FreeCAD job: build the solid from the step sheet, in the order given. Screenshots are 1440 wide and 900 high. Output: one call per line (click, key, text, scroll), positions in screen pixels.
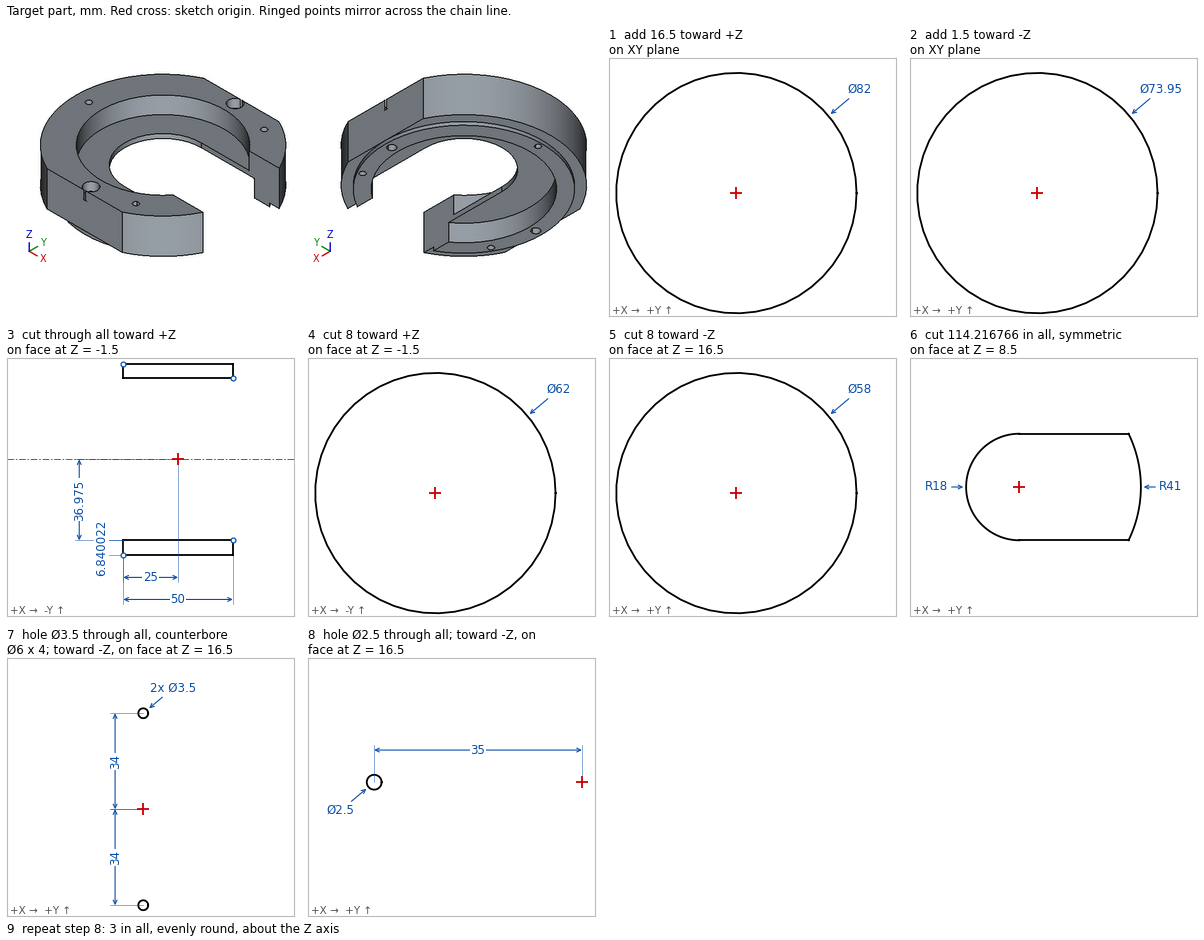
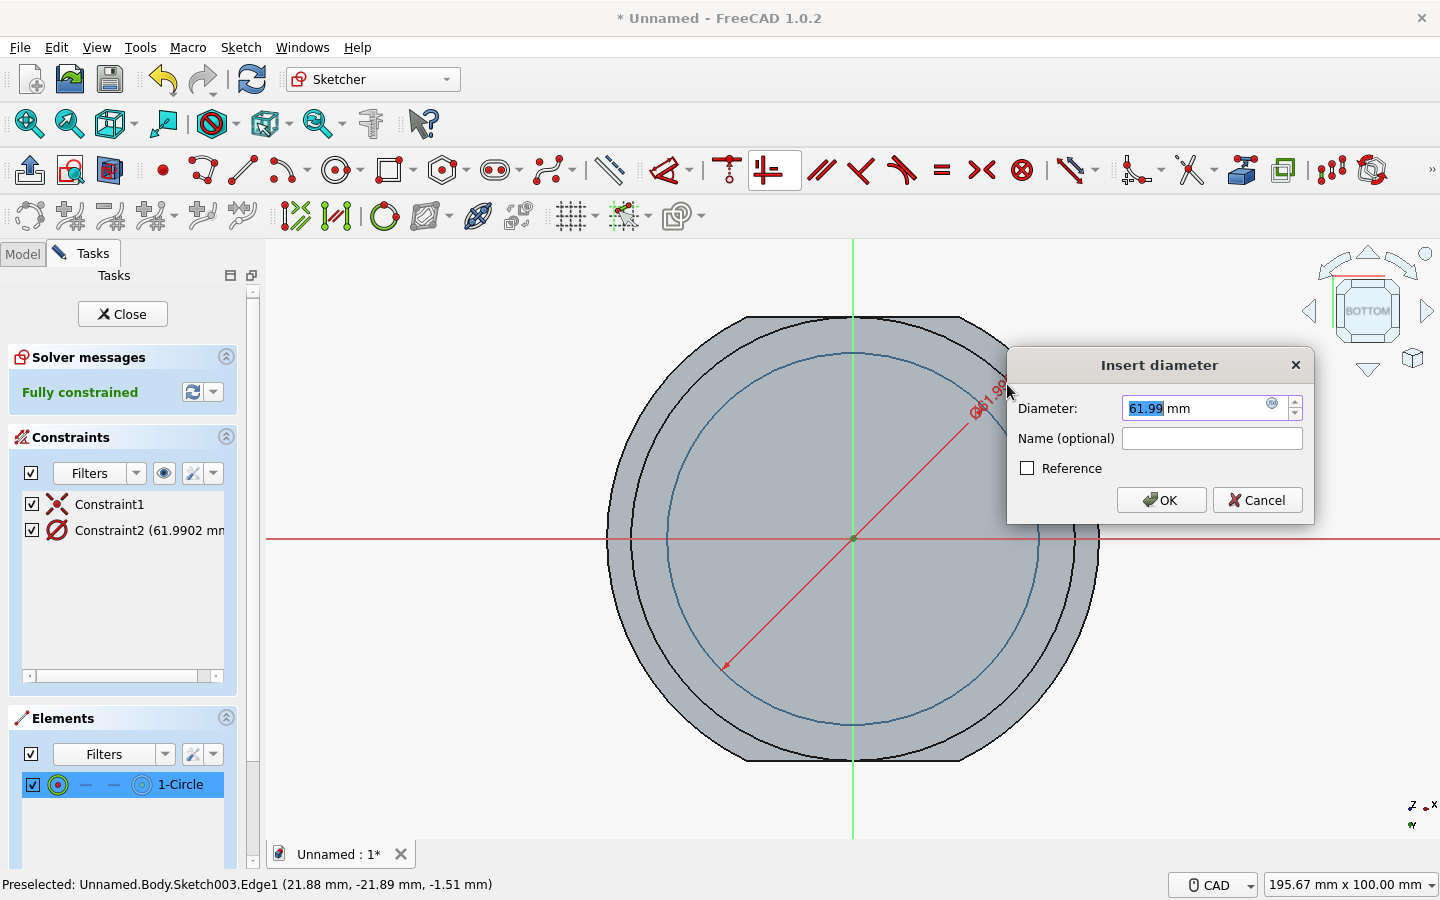
text(62)
key(Return)
key(Escape)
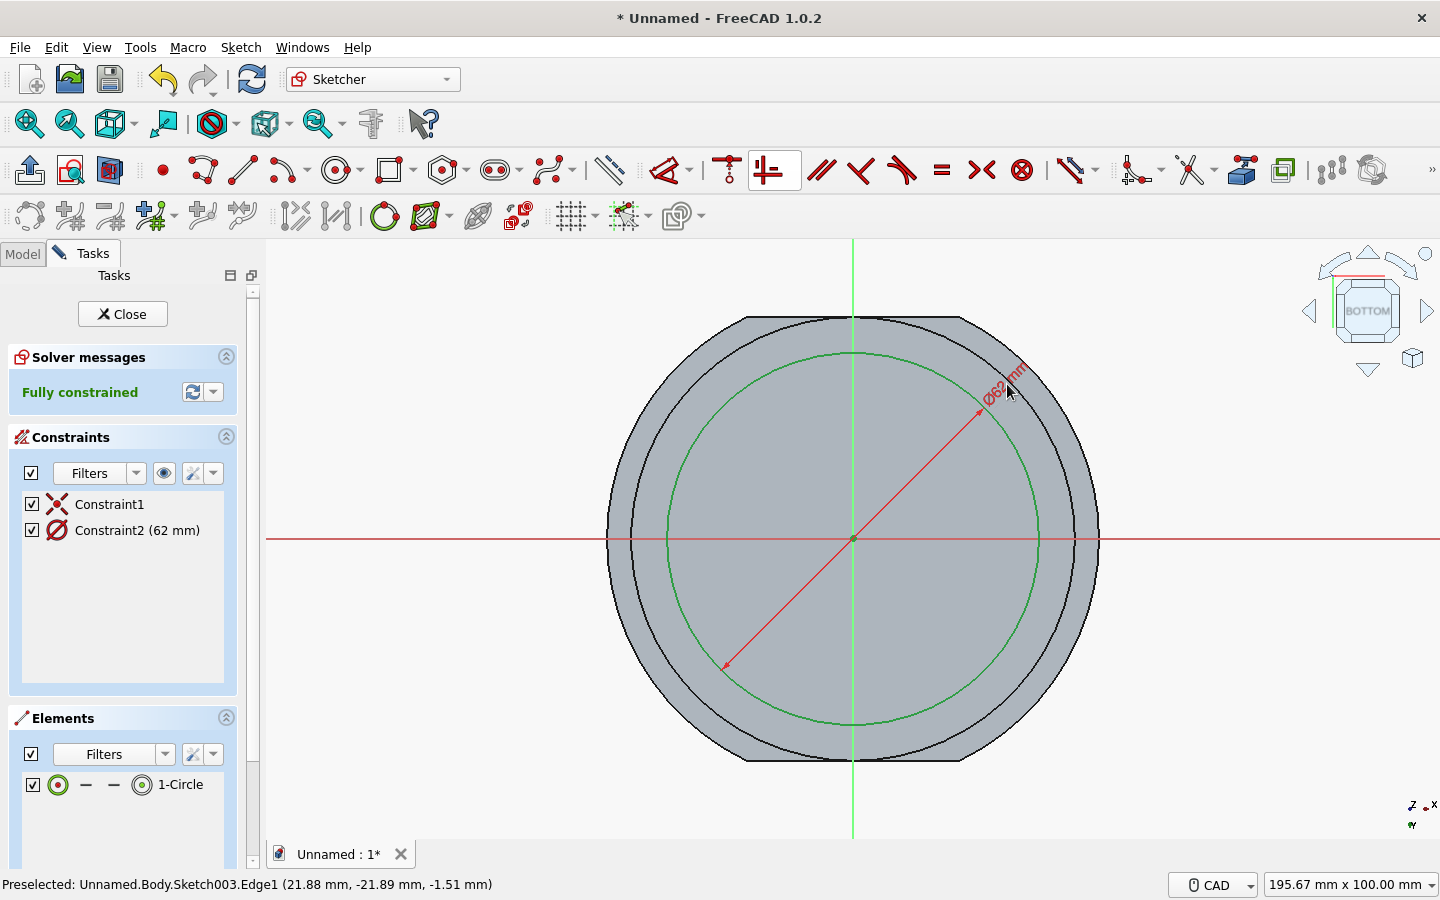
click(123, 314)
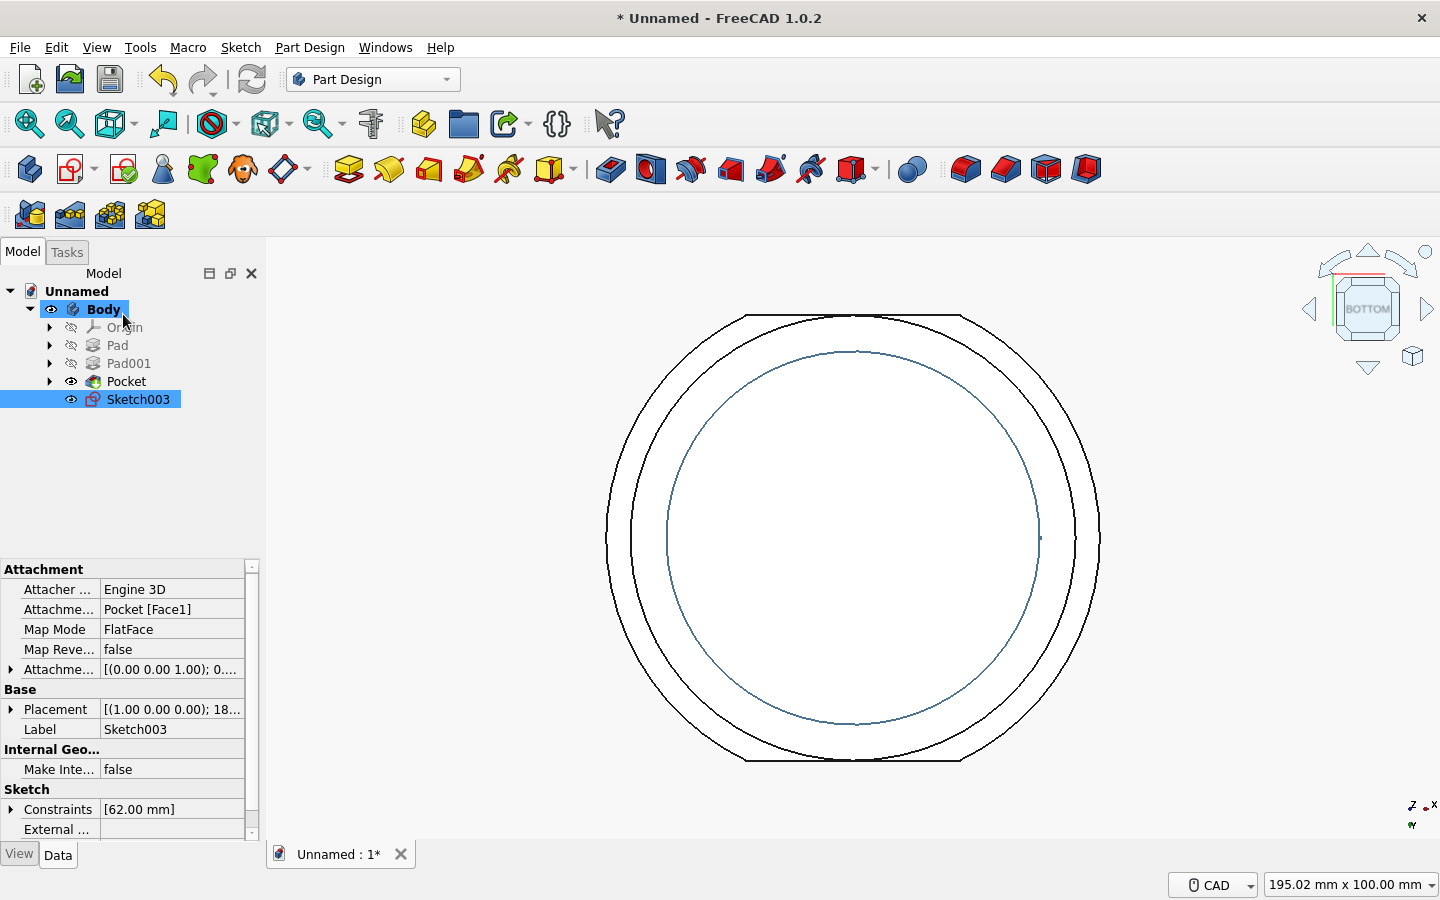
click(612, 170)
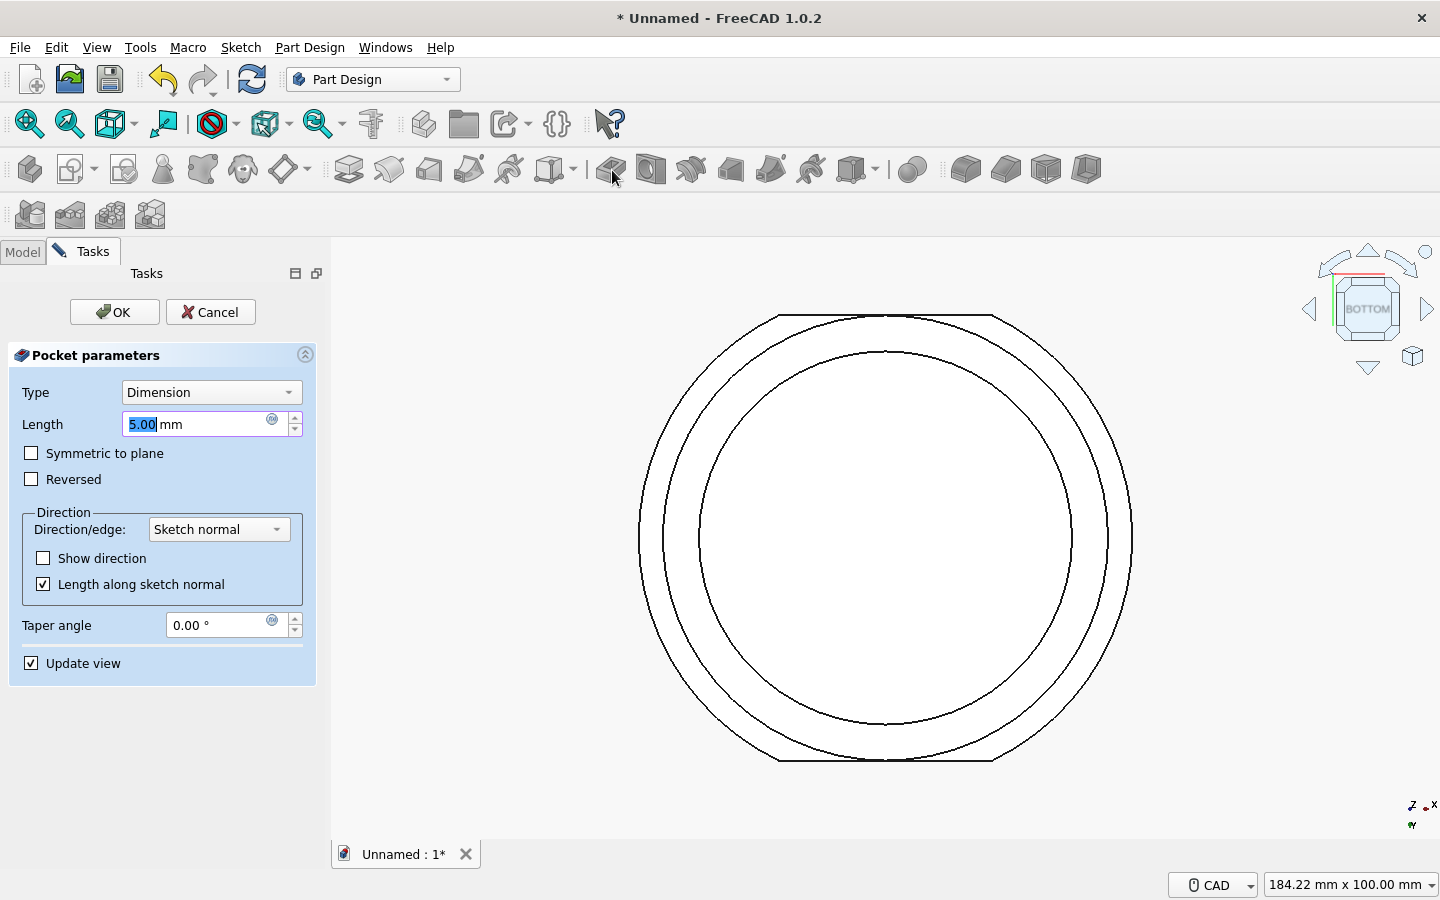
text(8)
key(Tab)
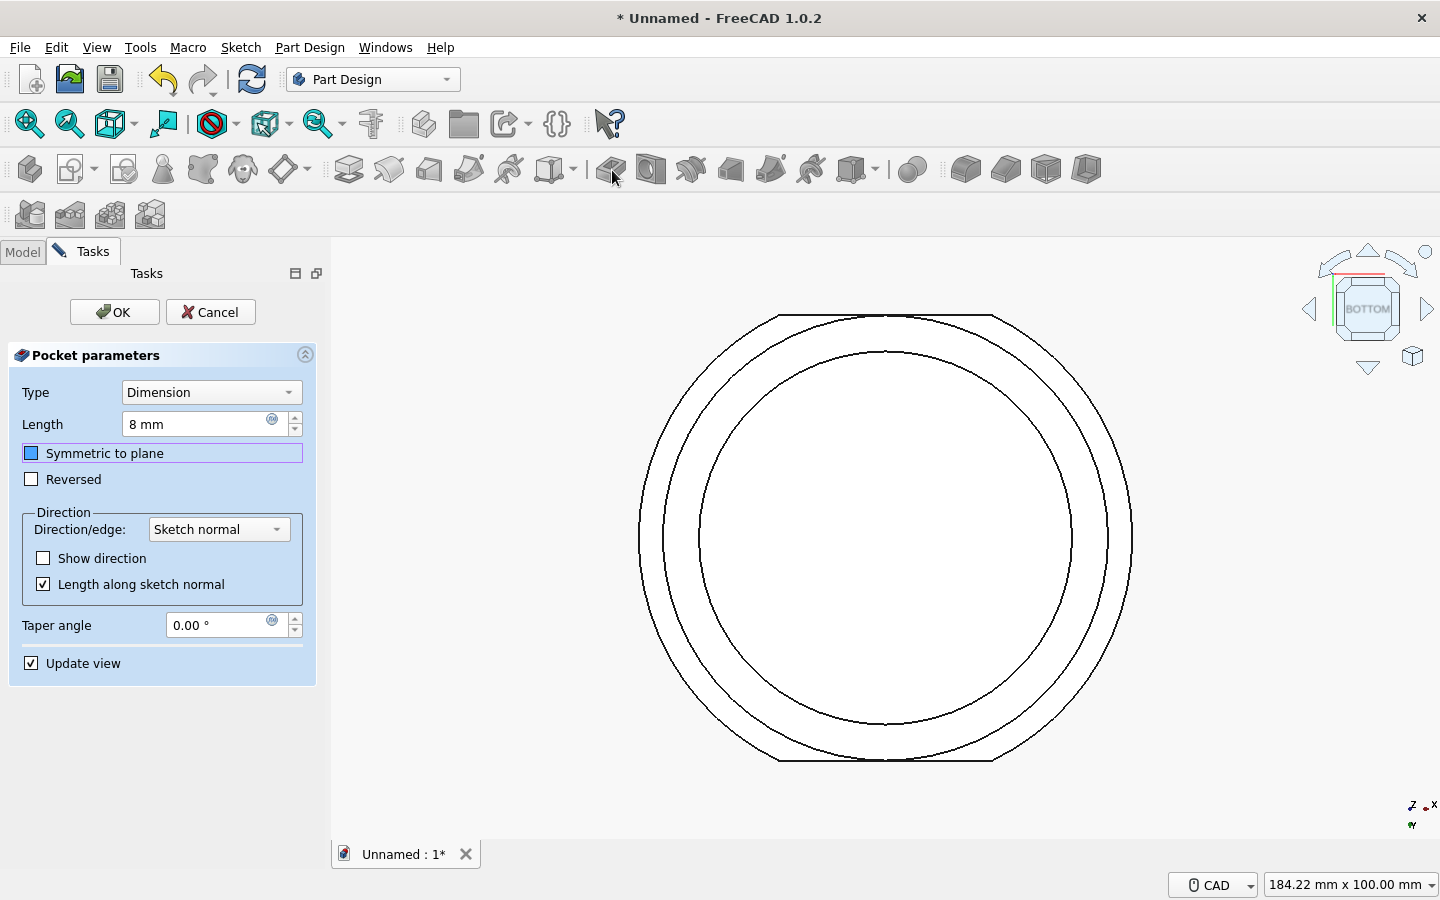
click(115, 312)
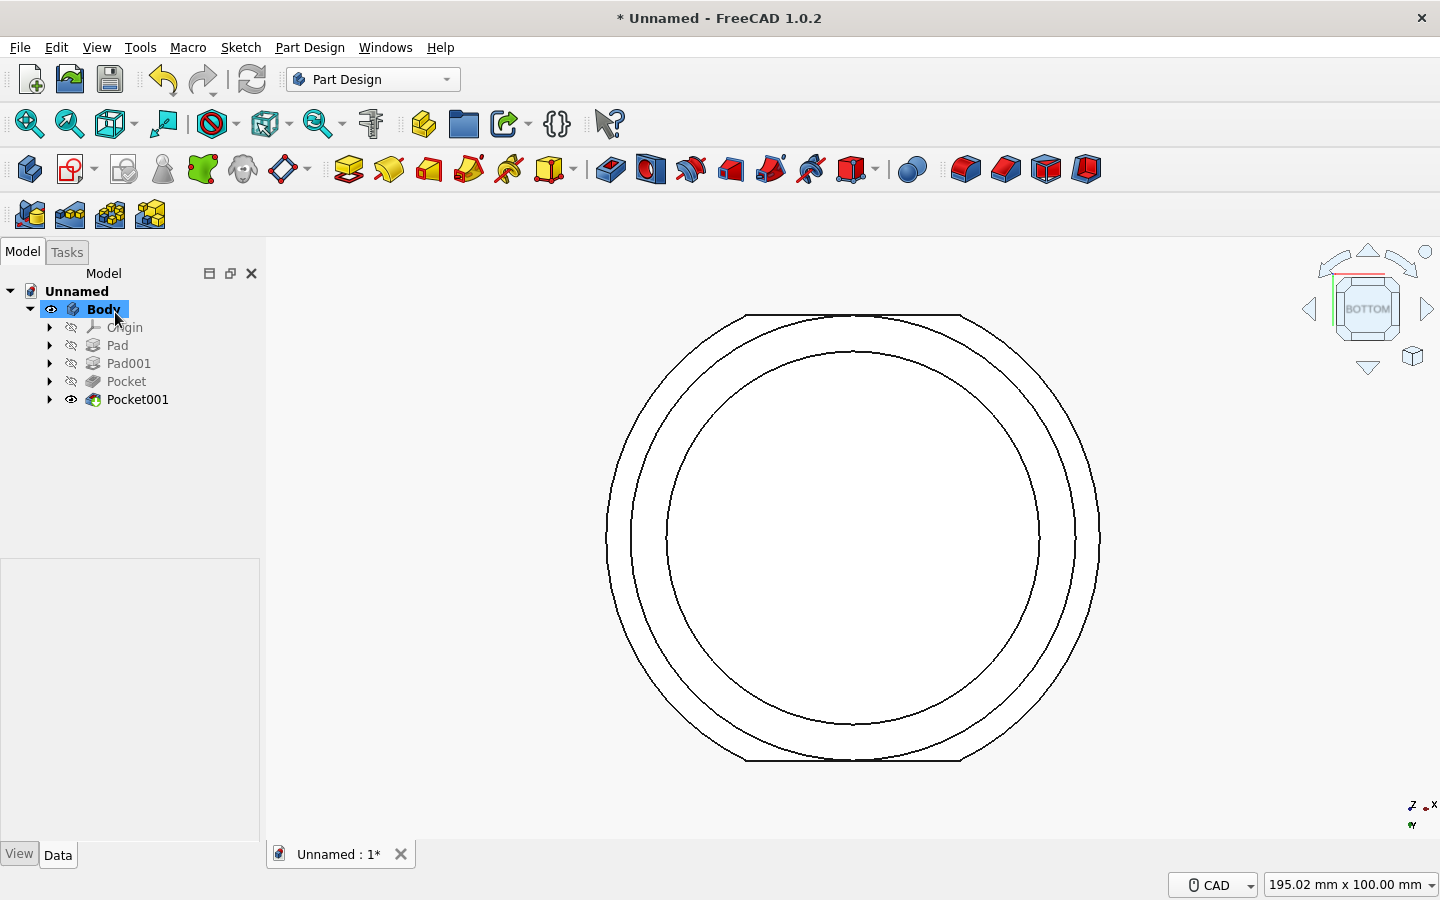
key(0)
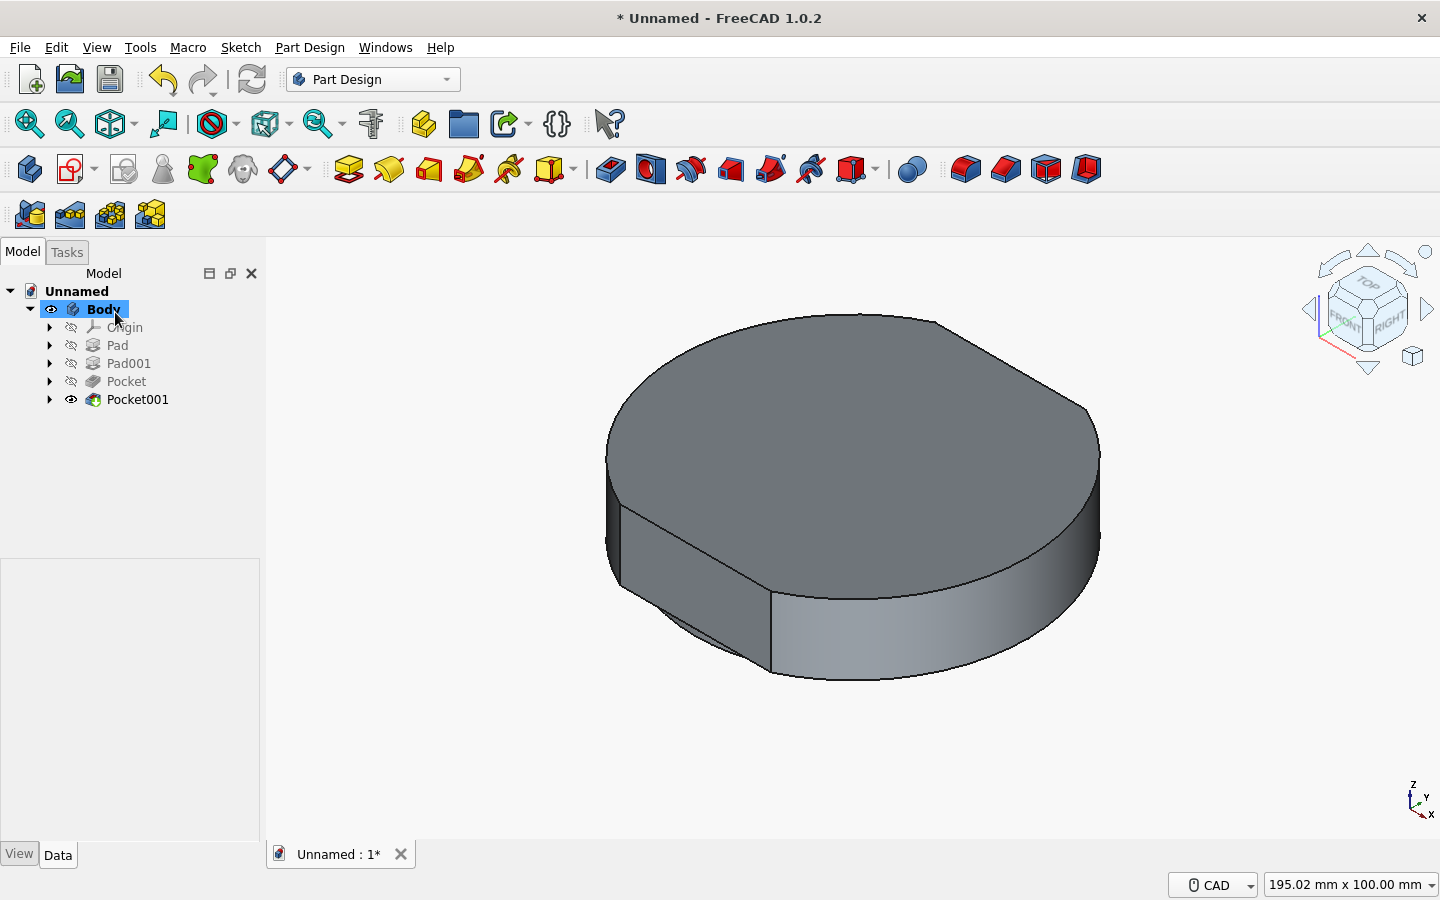
click(853, 456)